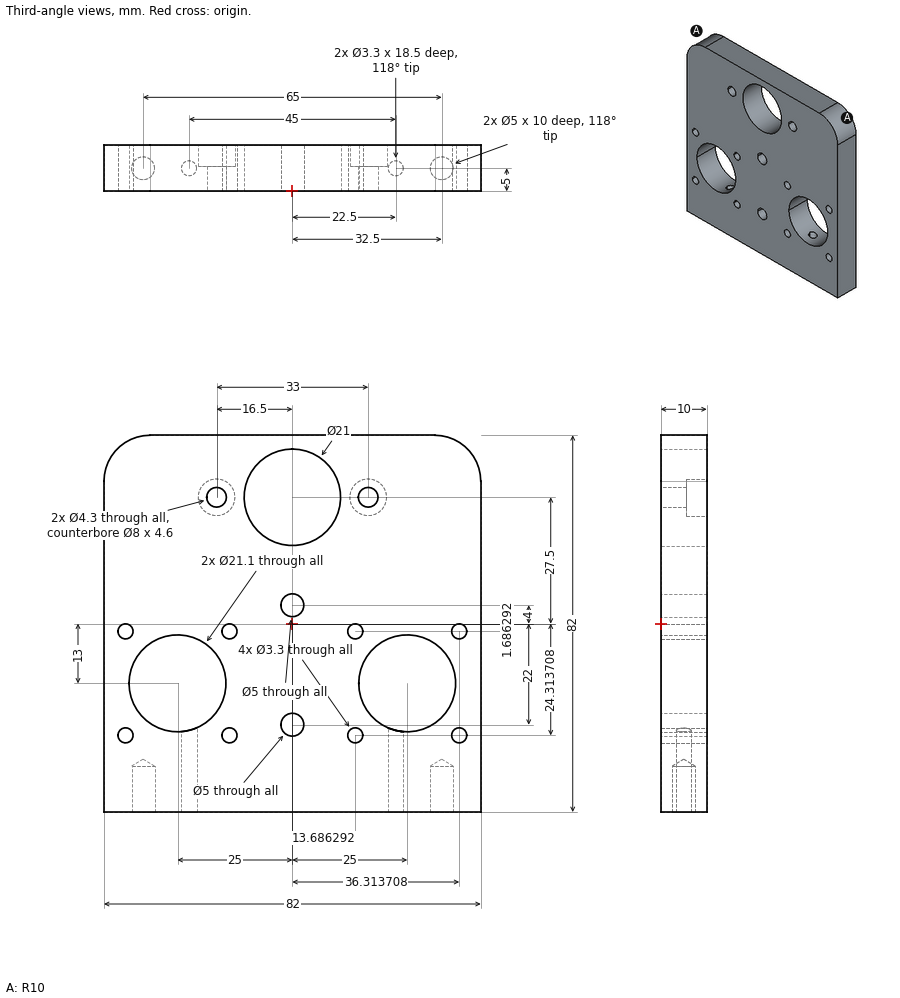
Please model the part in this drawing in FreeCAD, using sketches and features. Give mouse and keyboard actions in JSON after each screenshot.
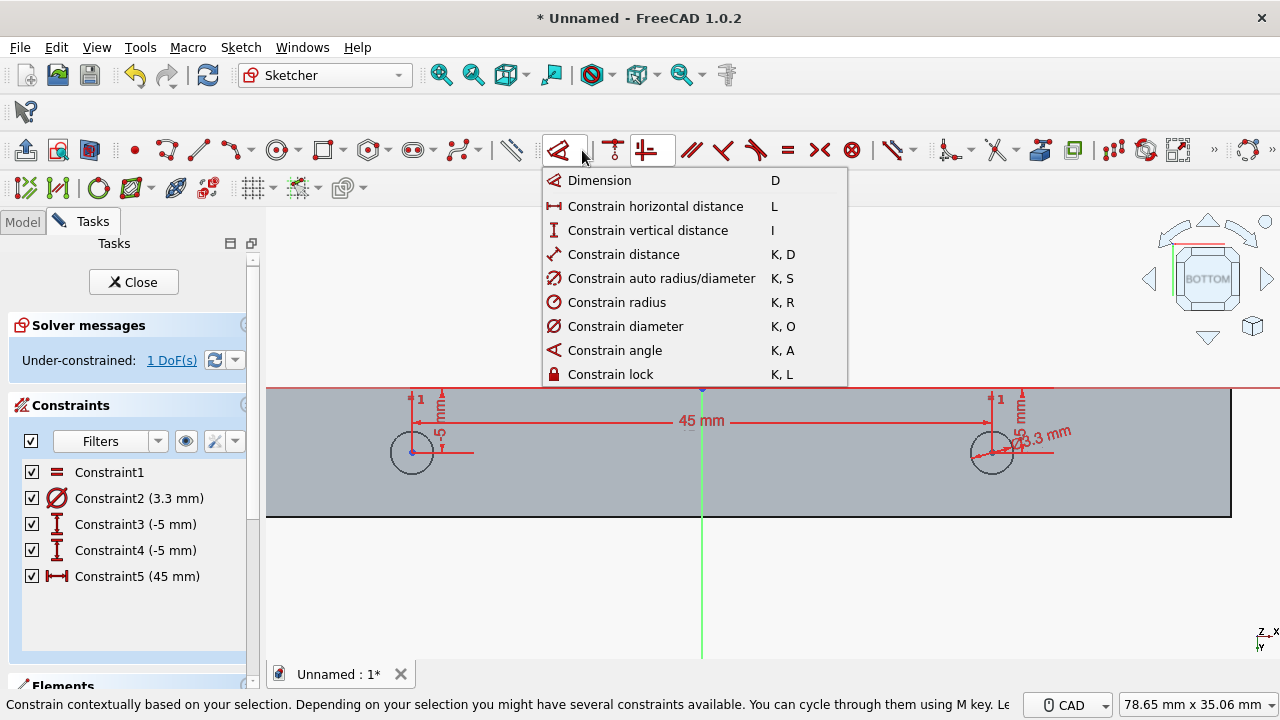
{"action": "left_click", "coordinate": [695, 206]}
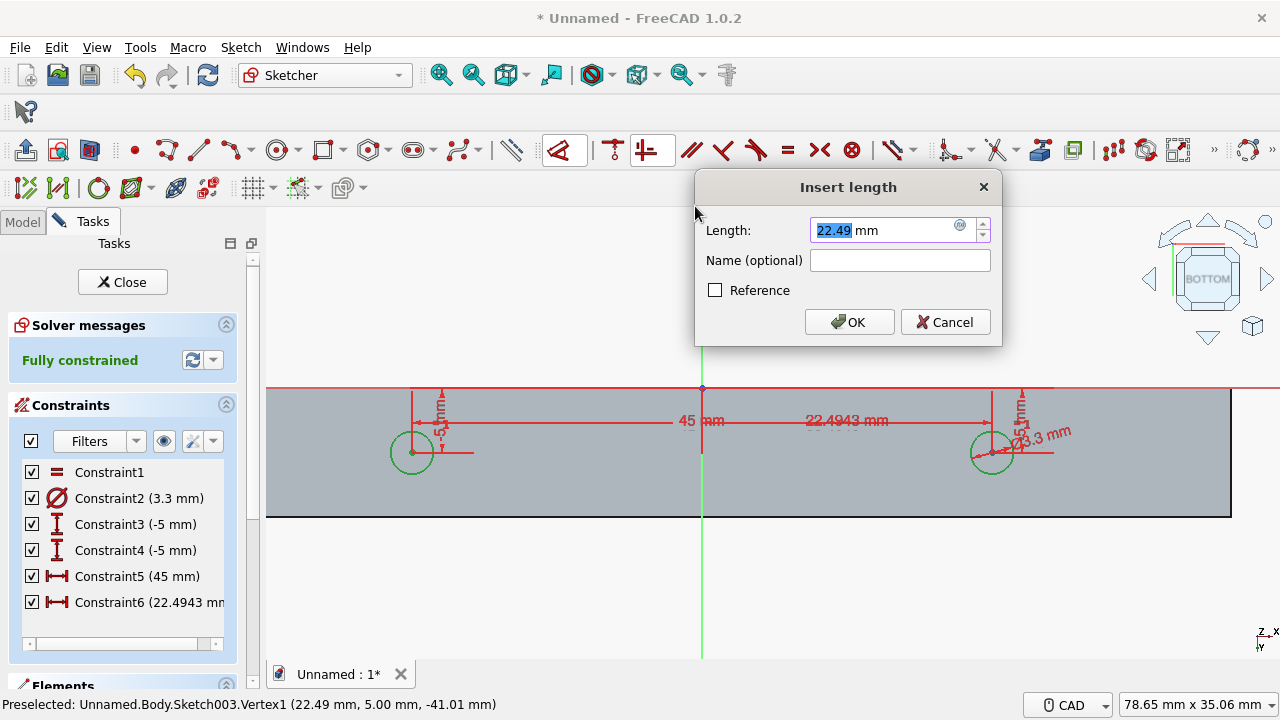
{"action": "type", "text": "22.5"}
{"action": "key", "text": "Return"}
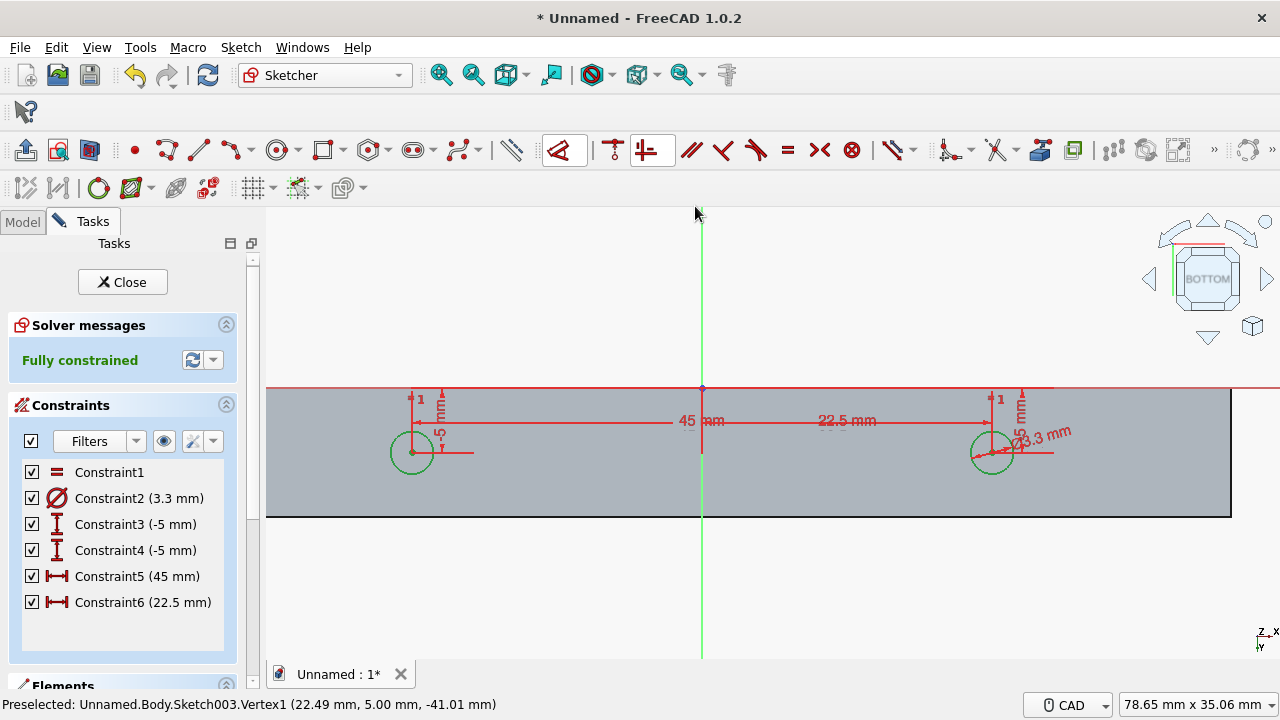
{"action": "left_click", "coordinate": [123, 282]}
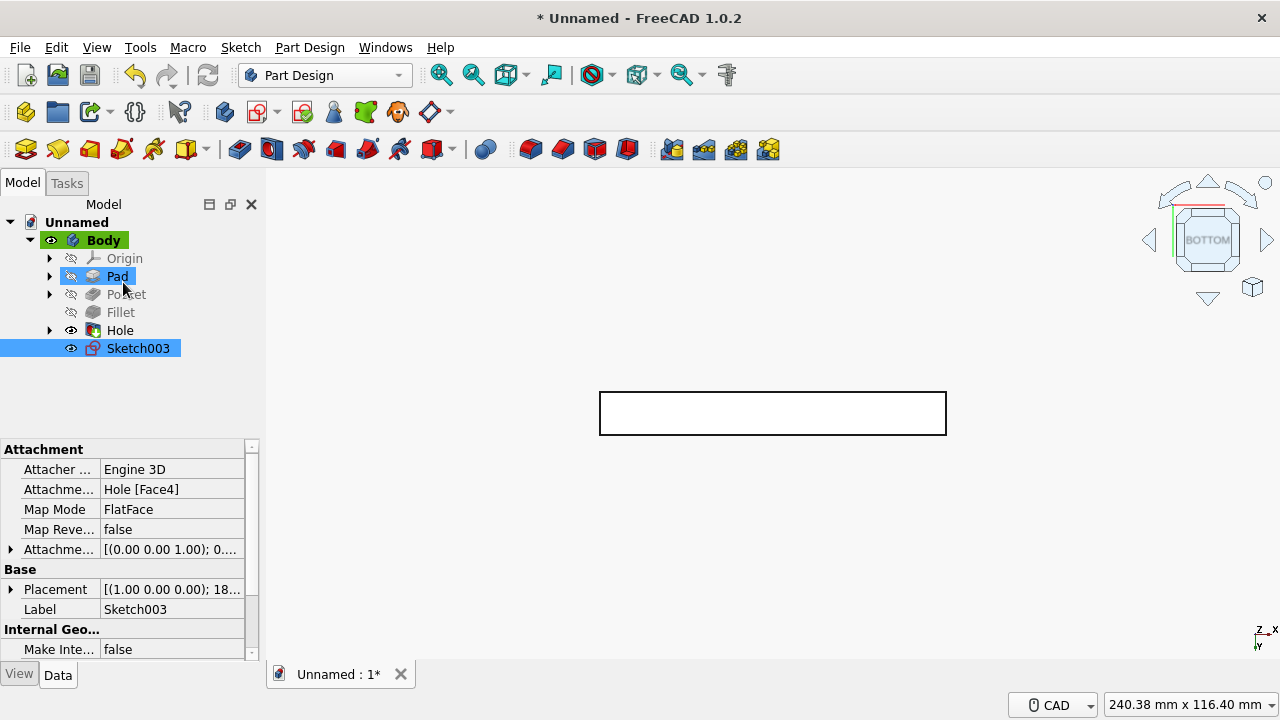
{"action": "left_click", "coordinate": [272, 150]}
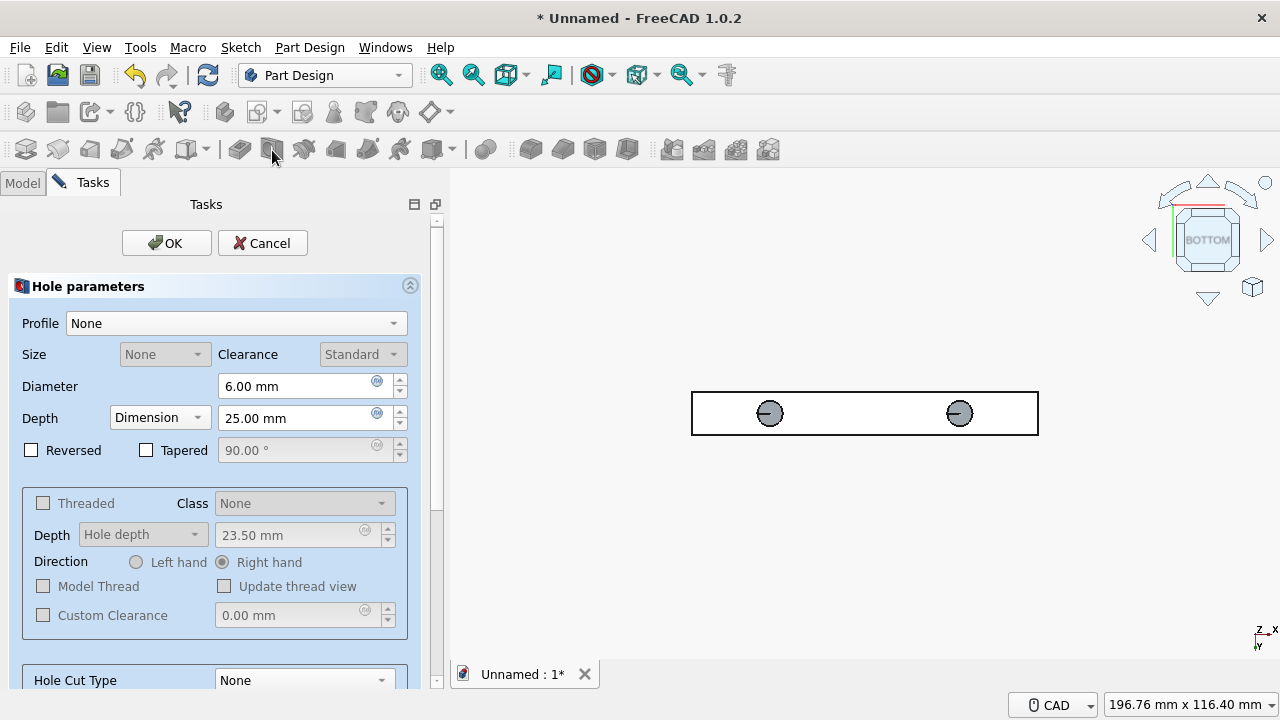
{"action": "triple_click", "coordinate": [305, 386]}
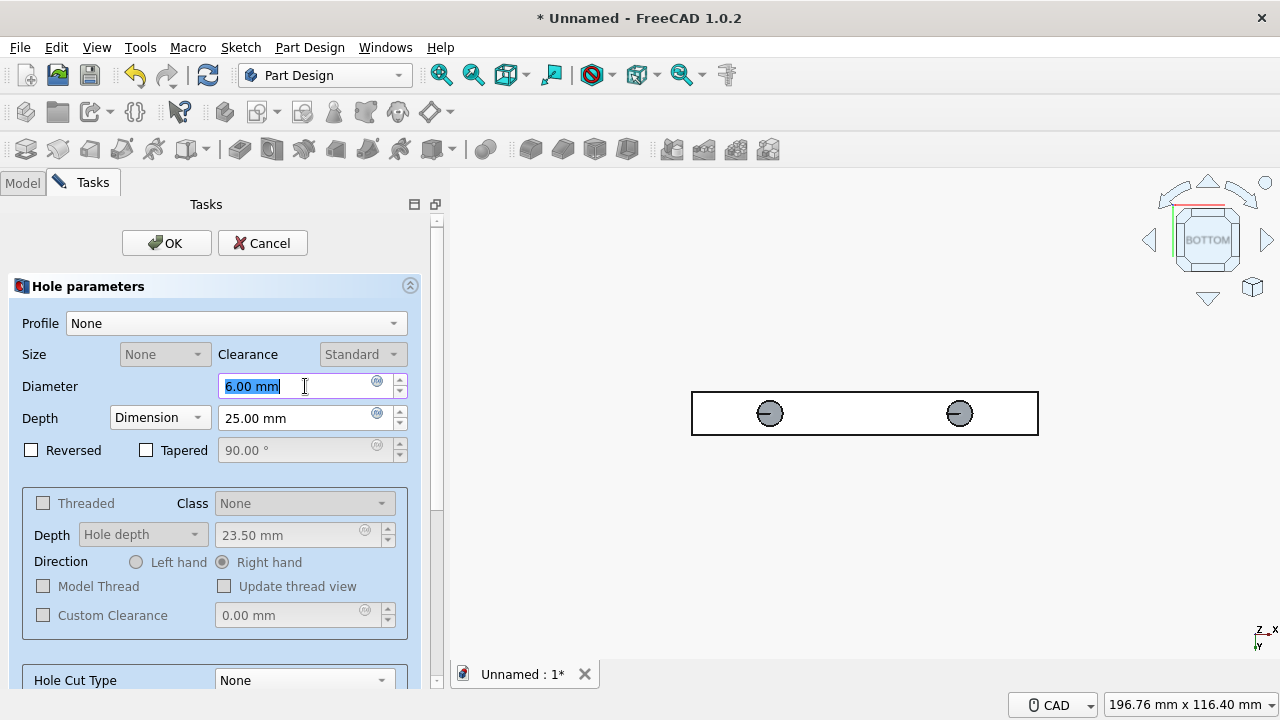
{"action": "type", "text": "3.3"}
{"action": "key", "text": "Tab"}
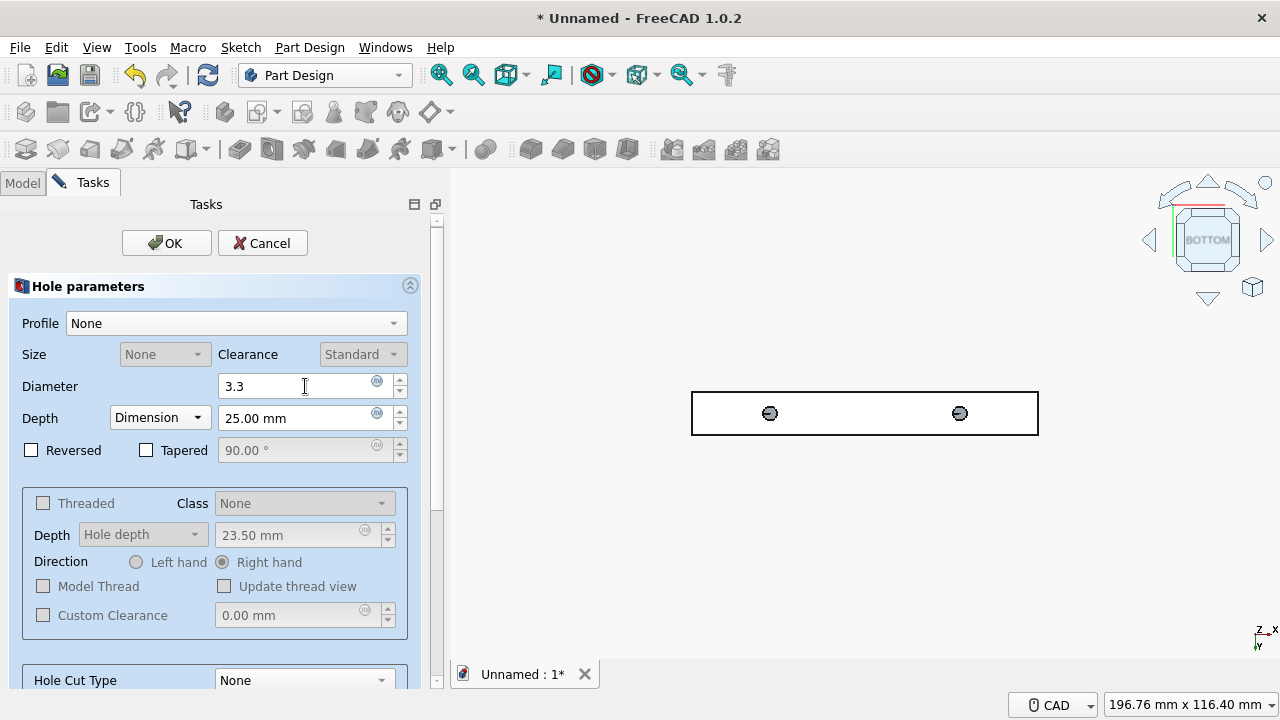
{"action": "triple_click", "coordinate": [305, 418]}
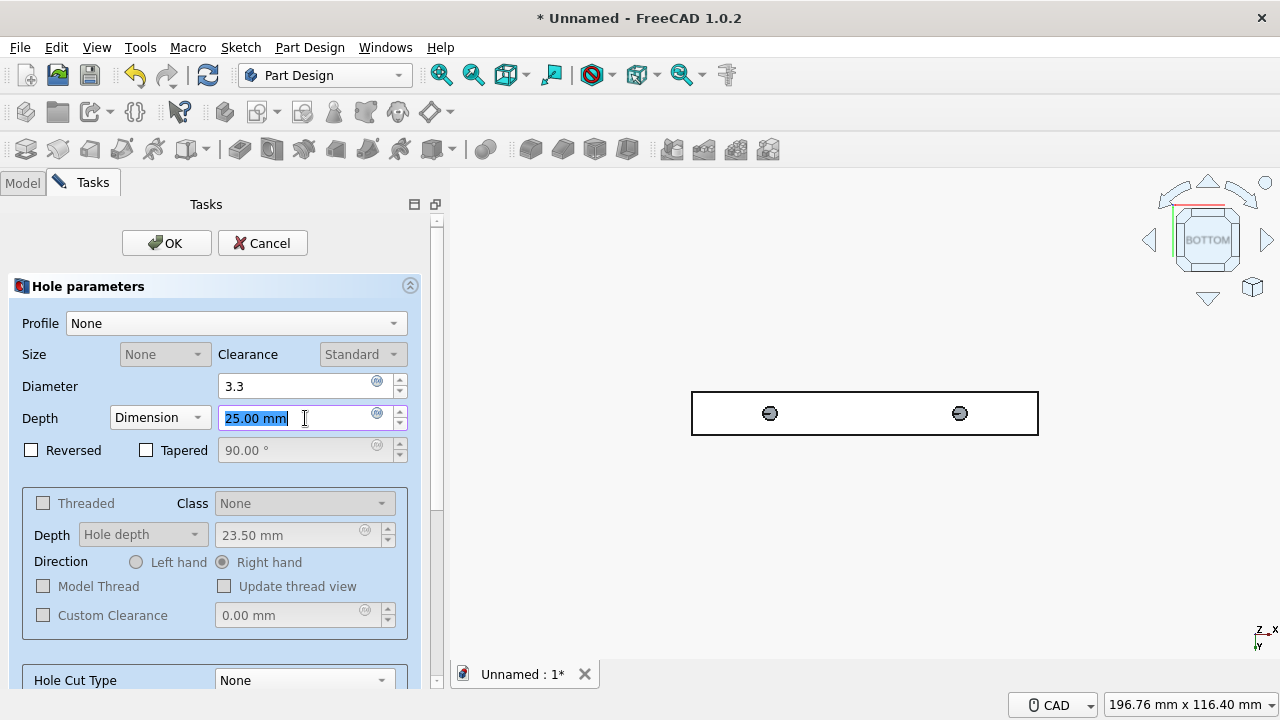
{"action": "type", "text": "18.5"}
{"action": "key", "text": "Tab"}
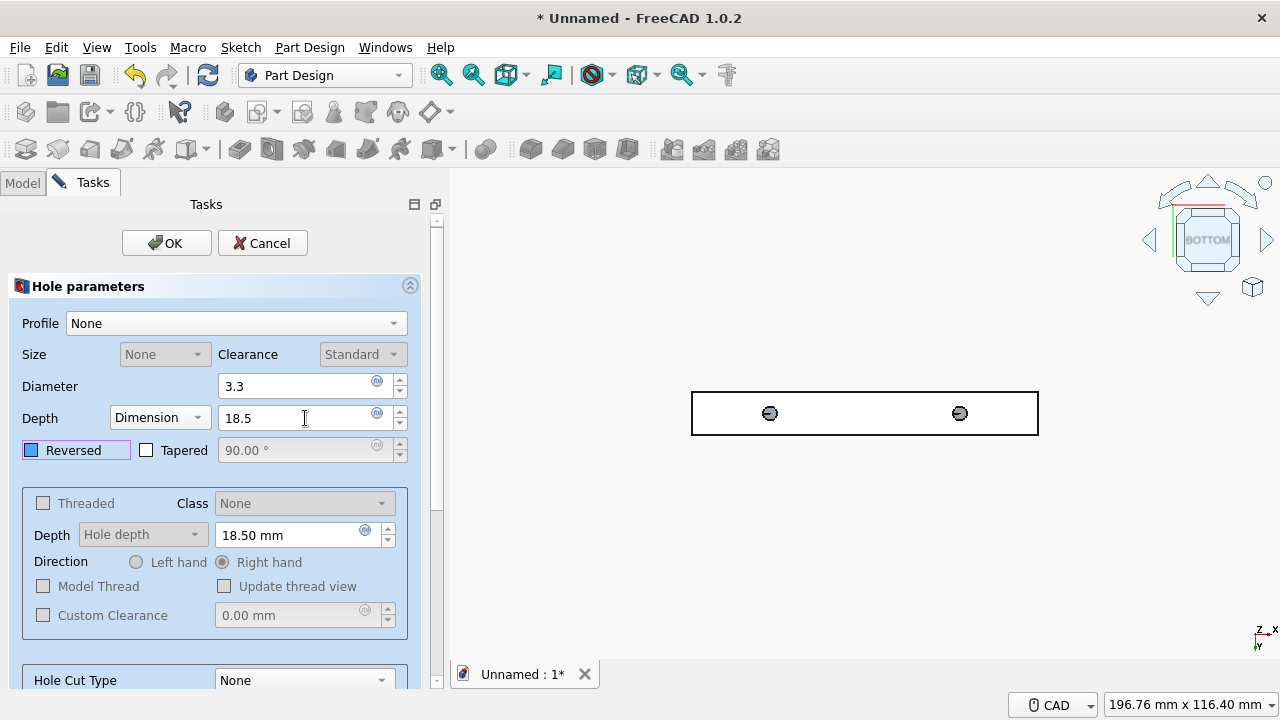
{"action": "left_click", "coordinate": [167, 243]}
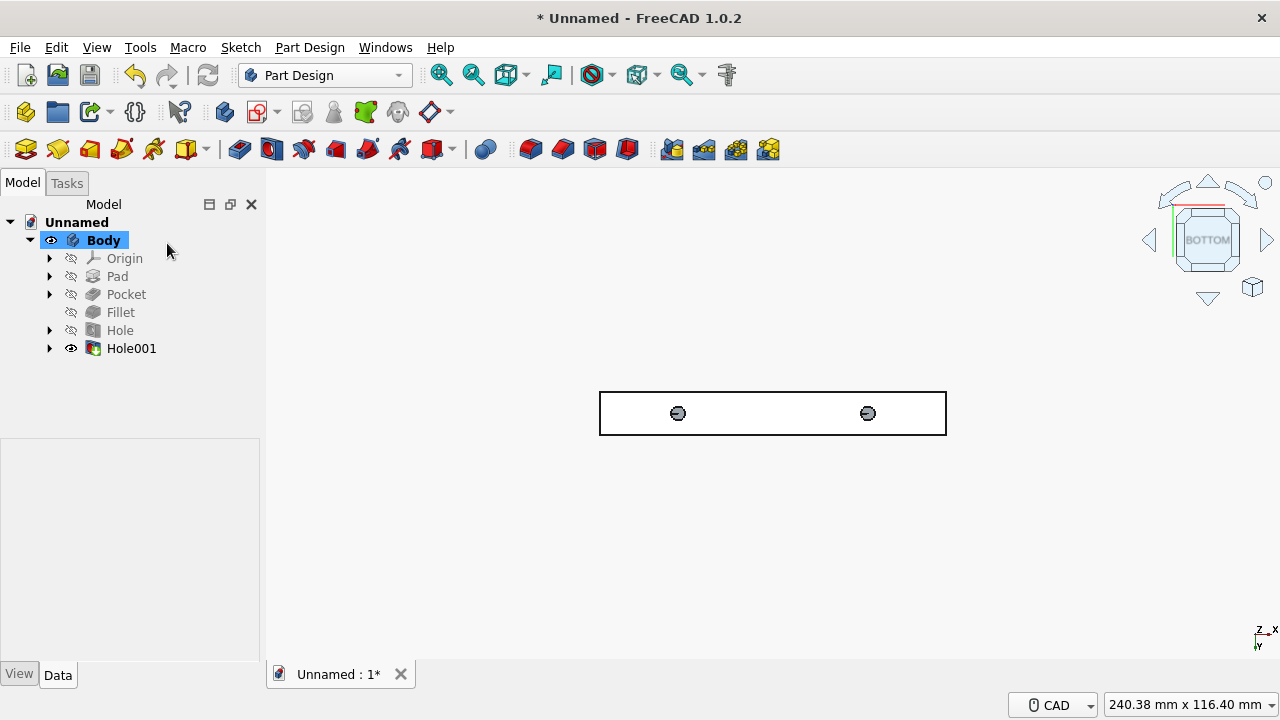
{"action": "left_click", "coordinate": [442, 76]}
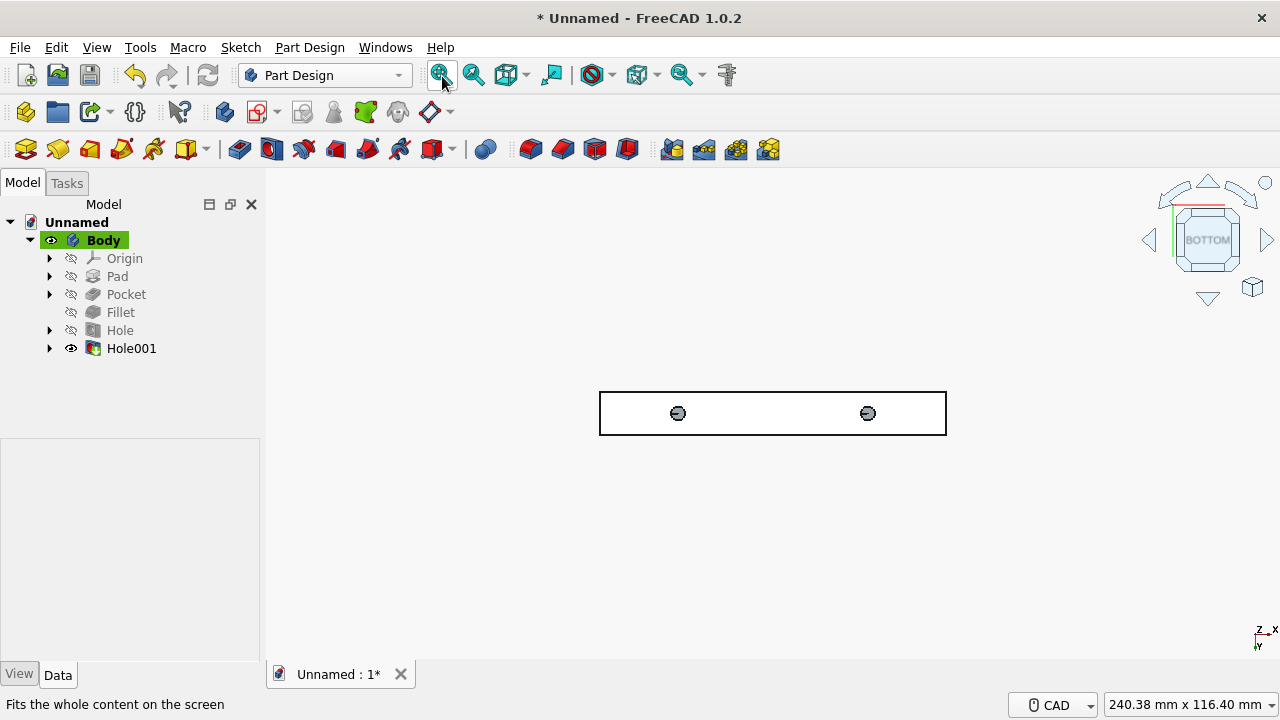
{"action": "key", "text": "4"}